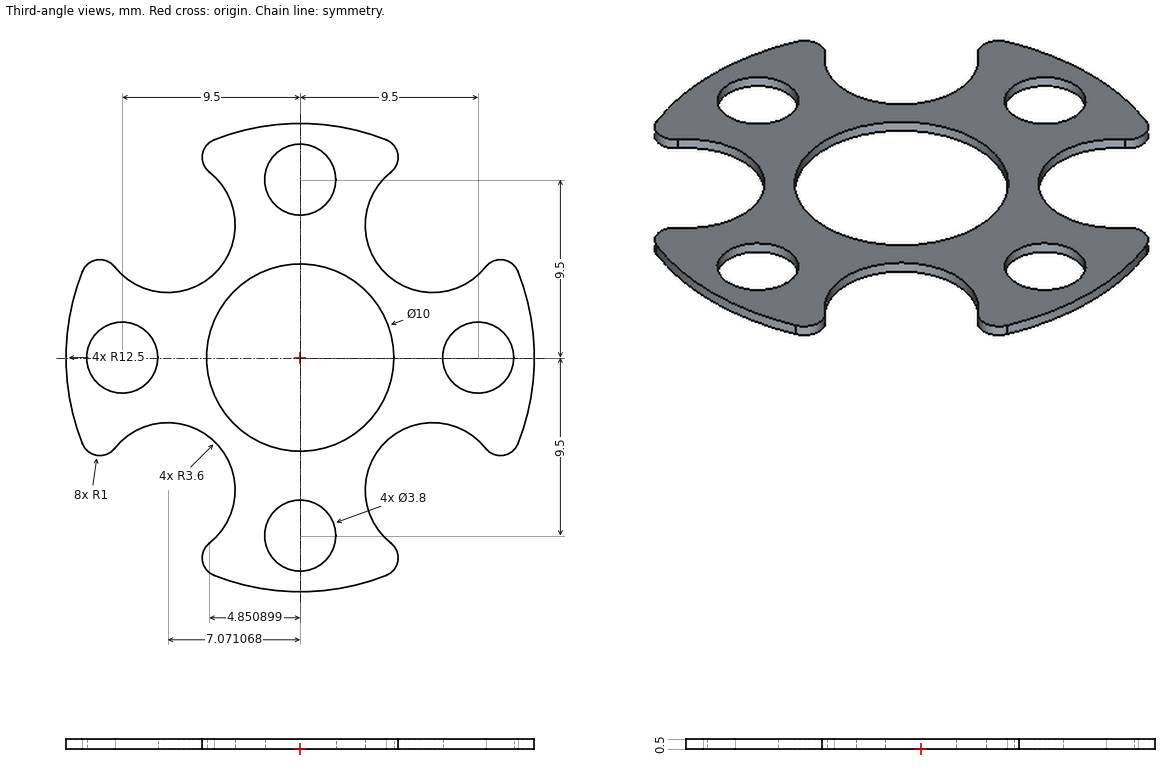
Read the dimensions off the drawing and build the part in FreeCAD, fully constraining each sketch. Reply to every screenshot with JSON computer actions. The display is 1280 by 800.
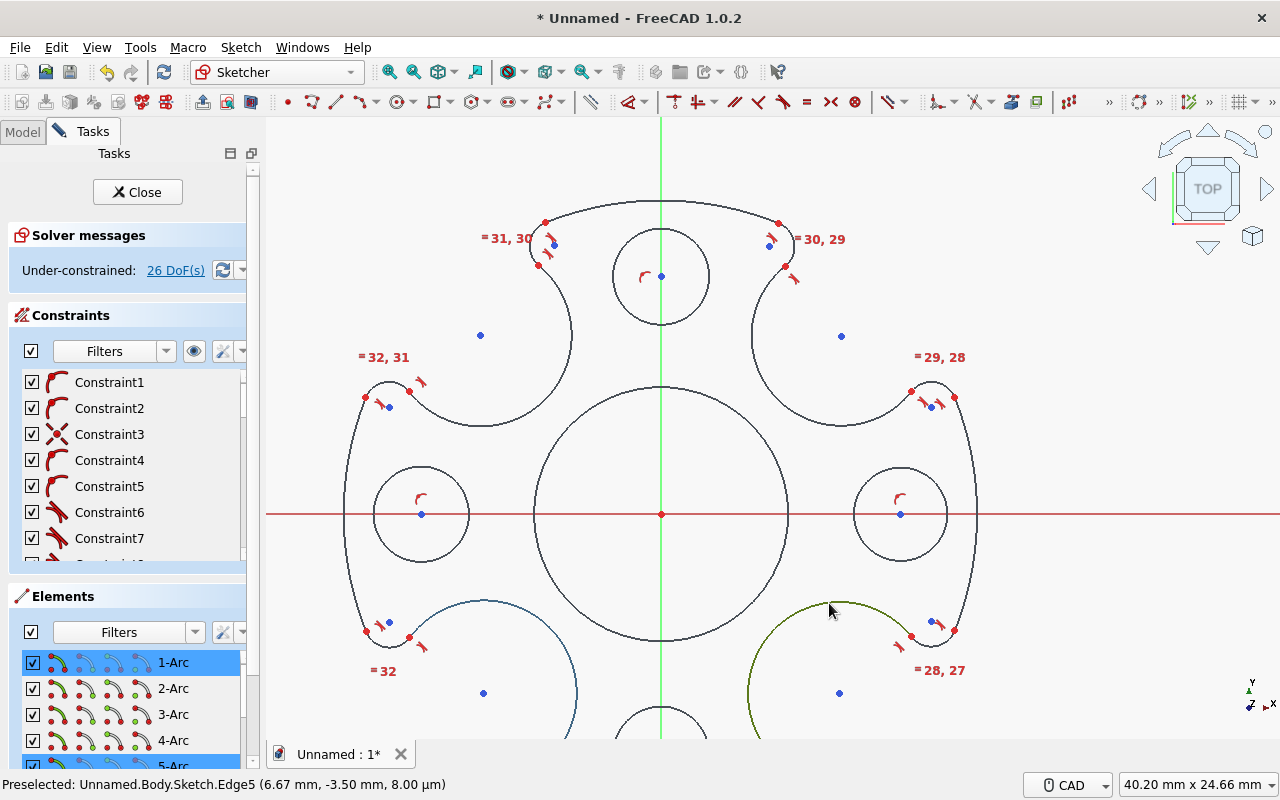
{"action": "left_click", "coordinate": [752, 347]}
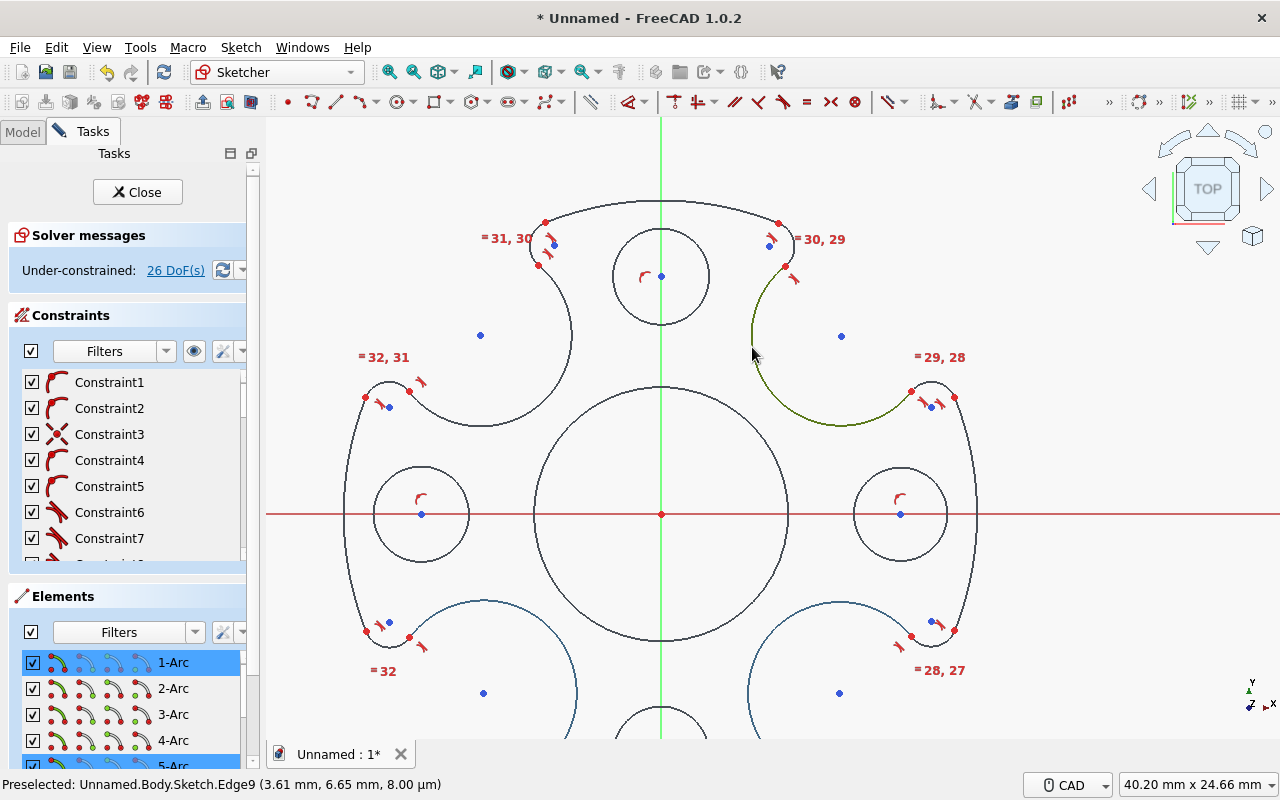
{"action": "left_click", "coordinate": [490, 426]}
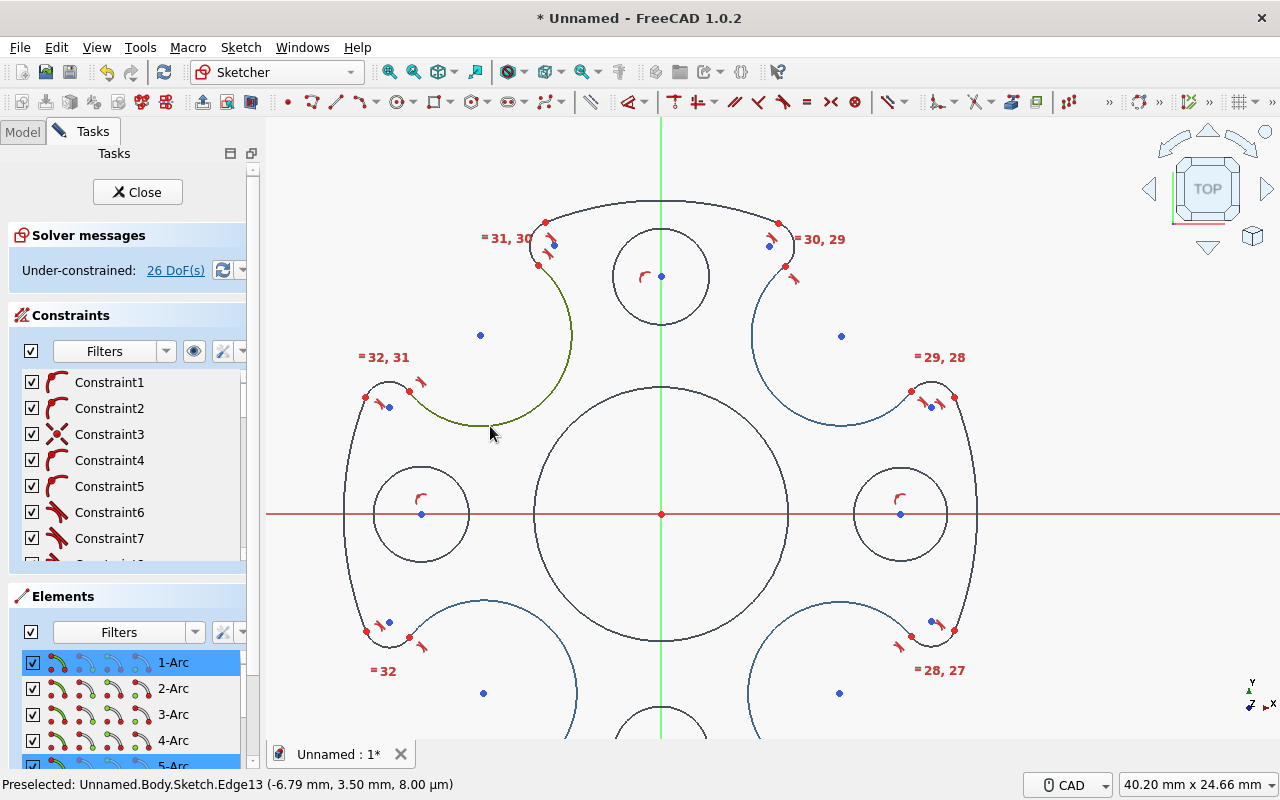
{"action": "key", "text": "e"}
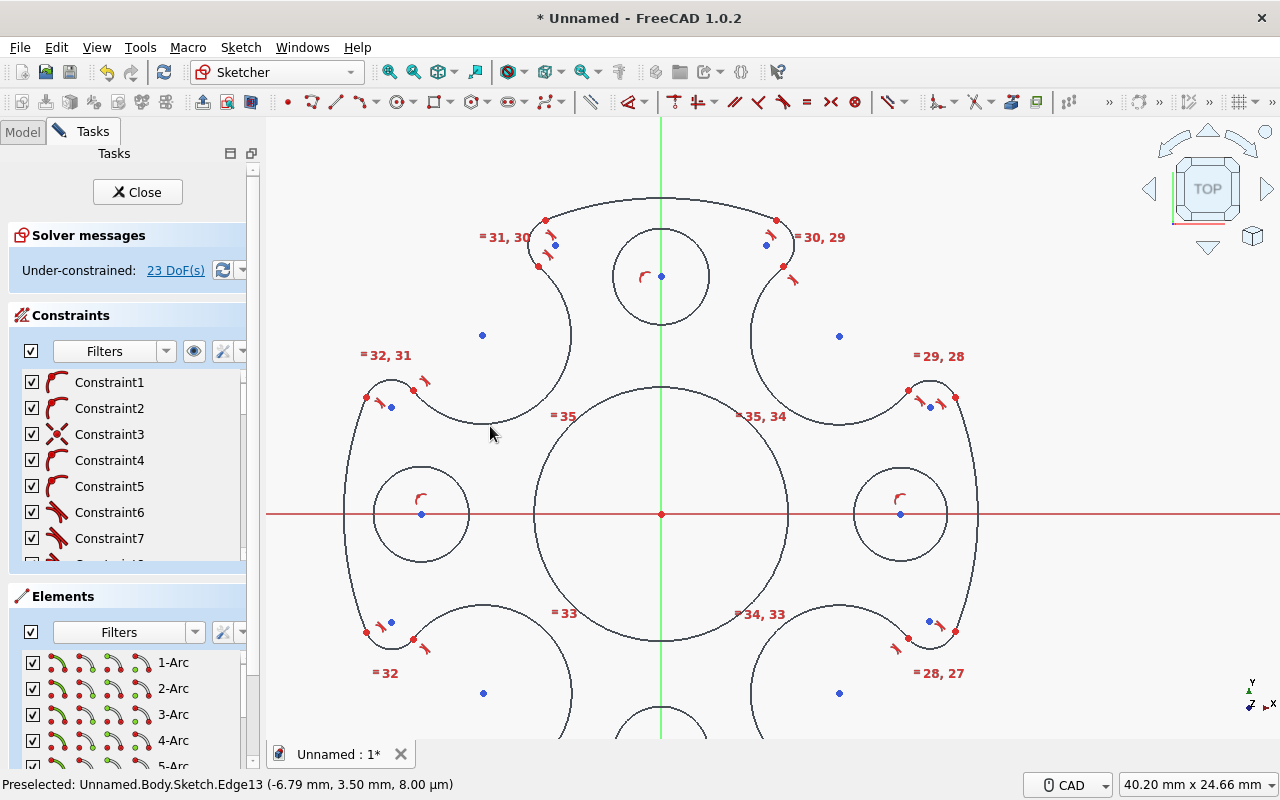
{"action": "scroll", "coordinate": [793, 253], "scroll_direction": "down", "scroll_amount": 2}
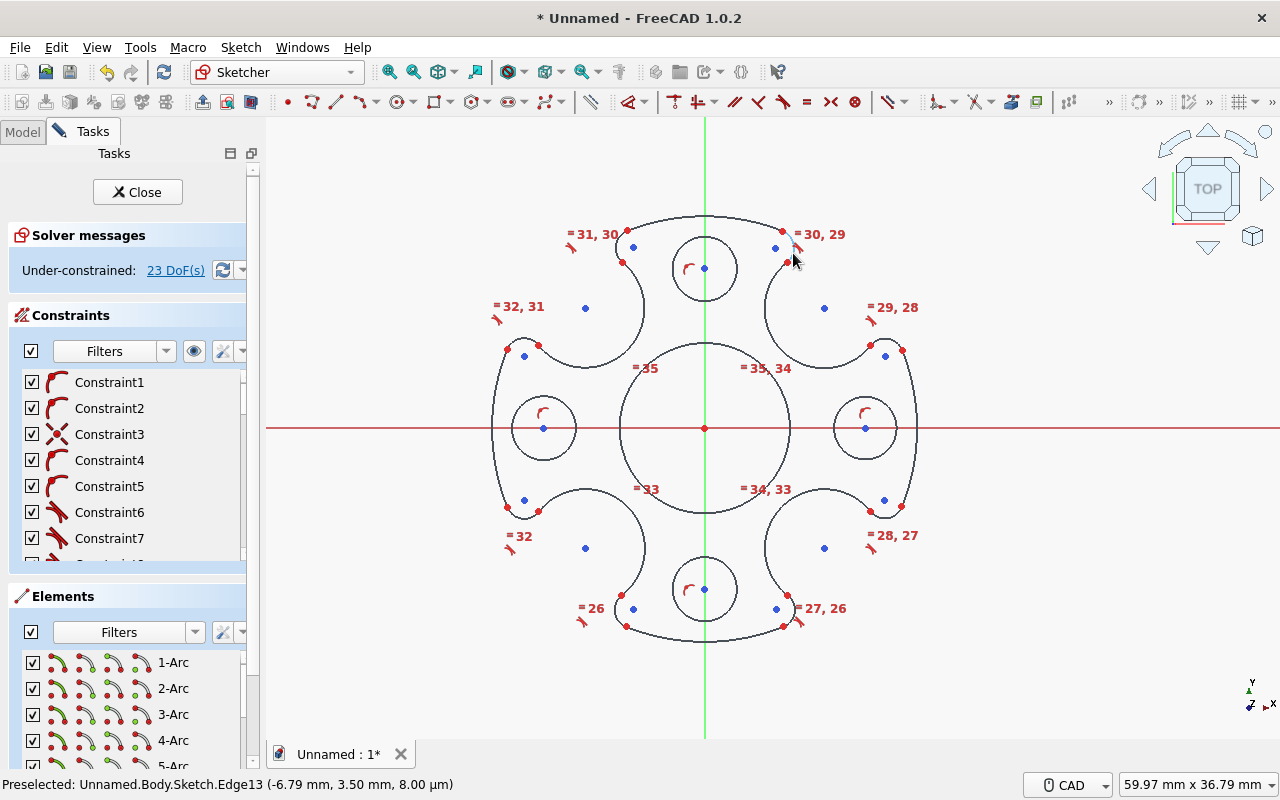
{"action": "left_click", "coordinate": [673, 639]}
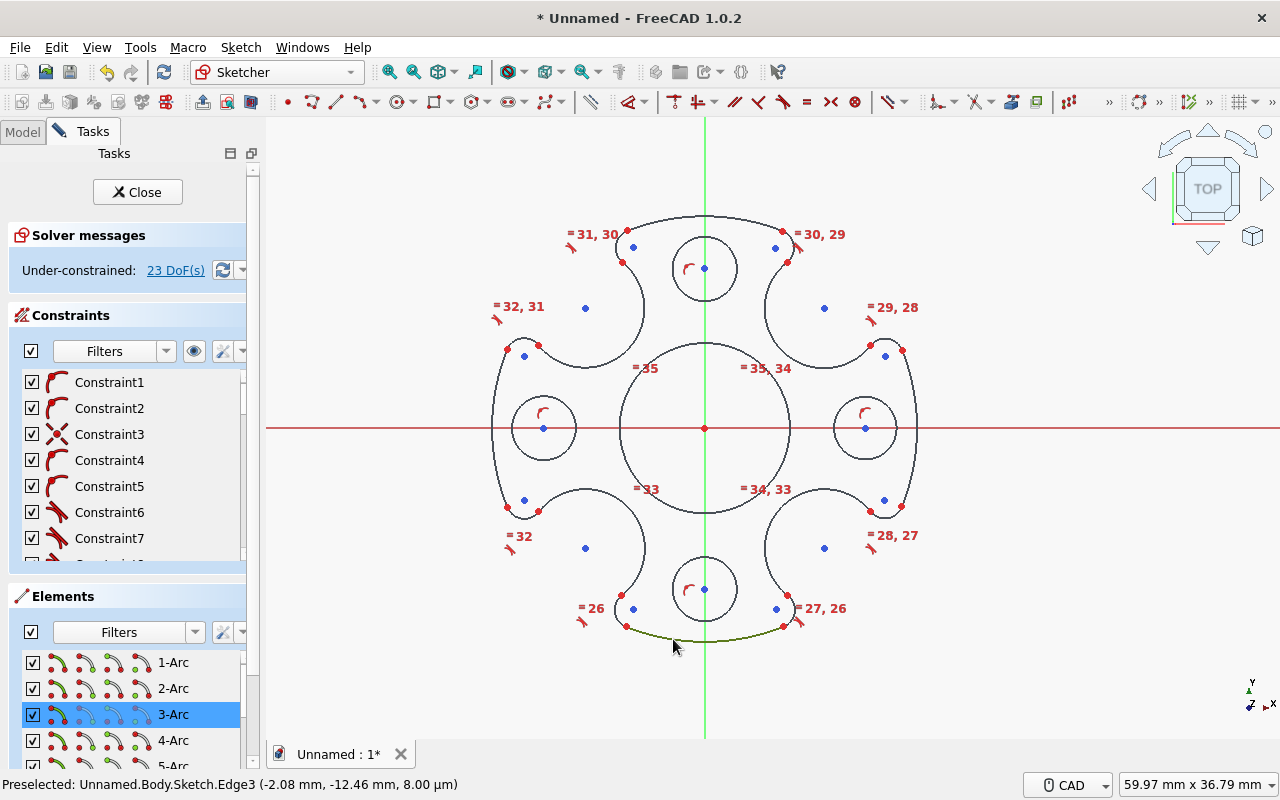
{"action": "left_click", "coordinate": [915, 460]}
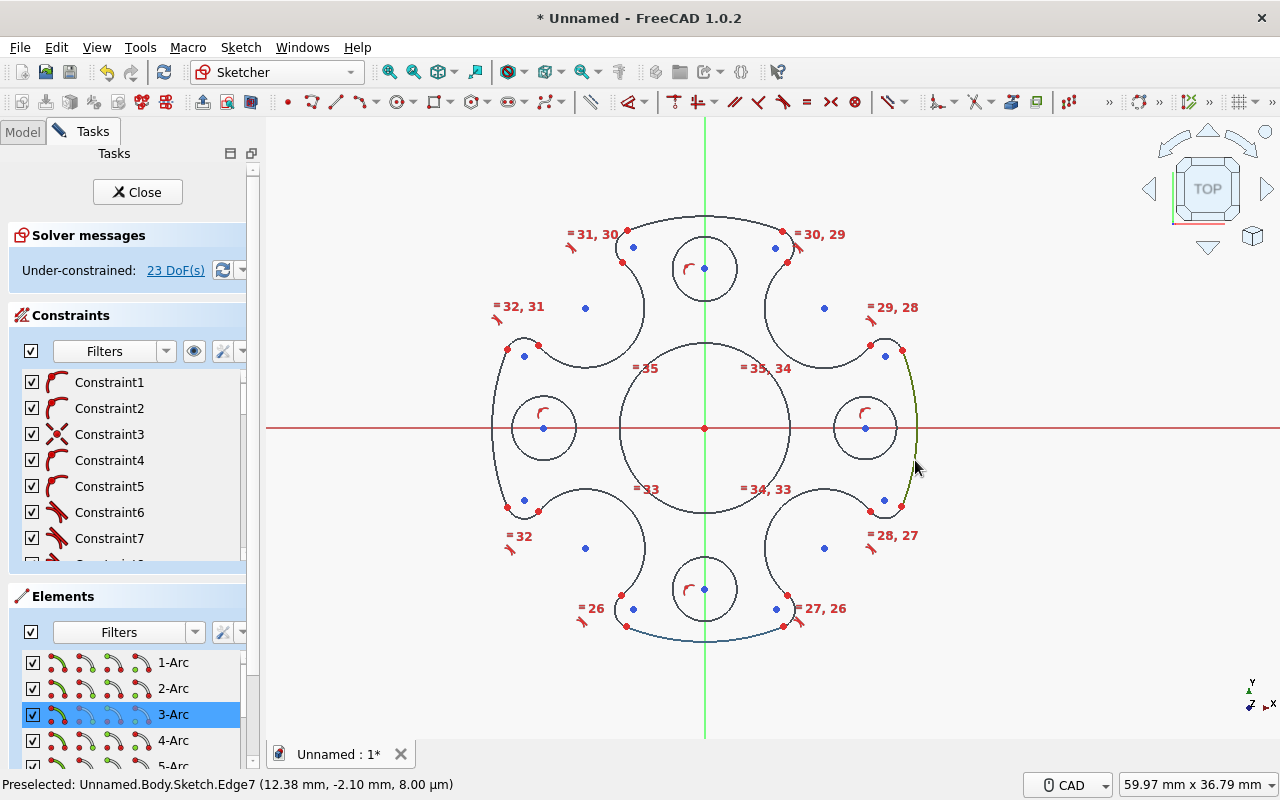
{"action": "left_click", "coordinate": [736, 219]}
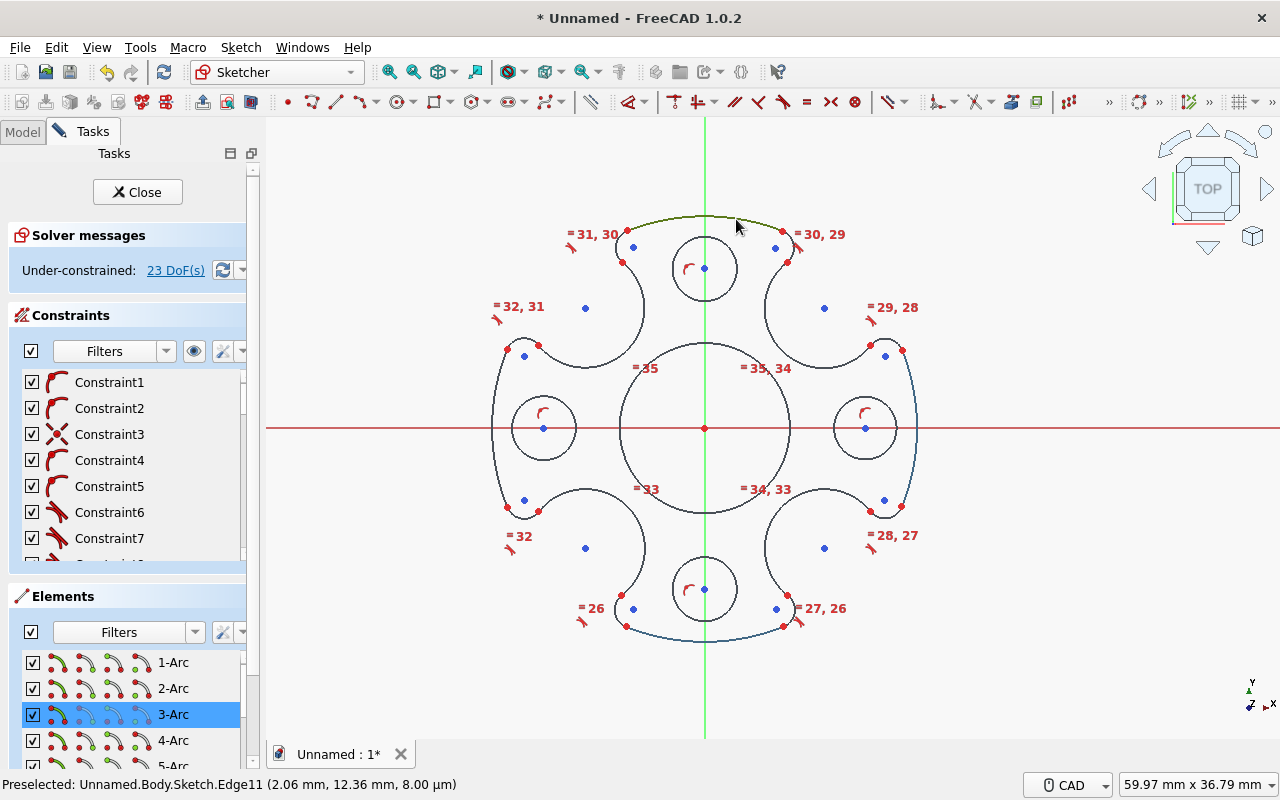
{"action": "left_click", "coordinate": [495, 396]}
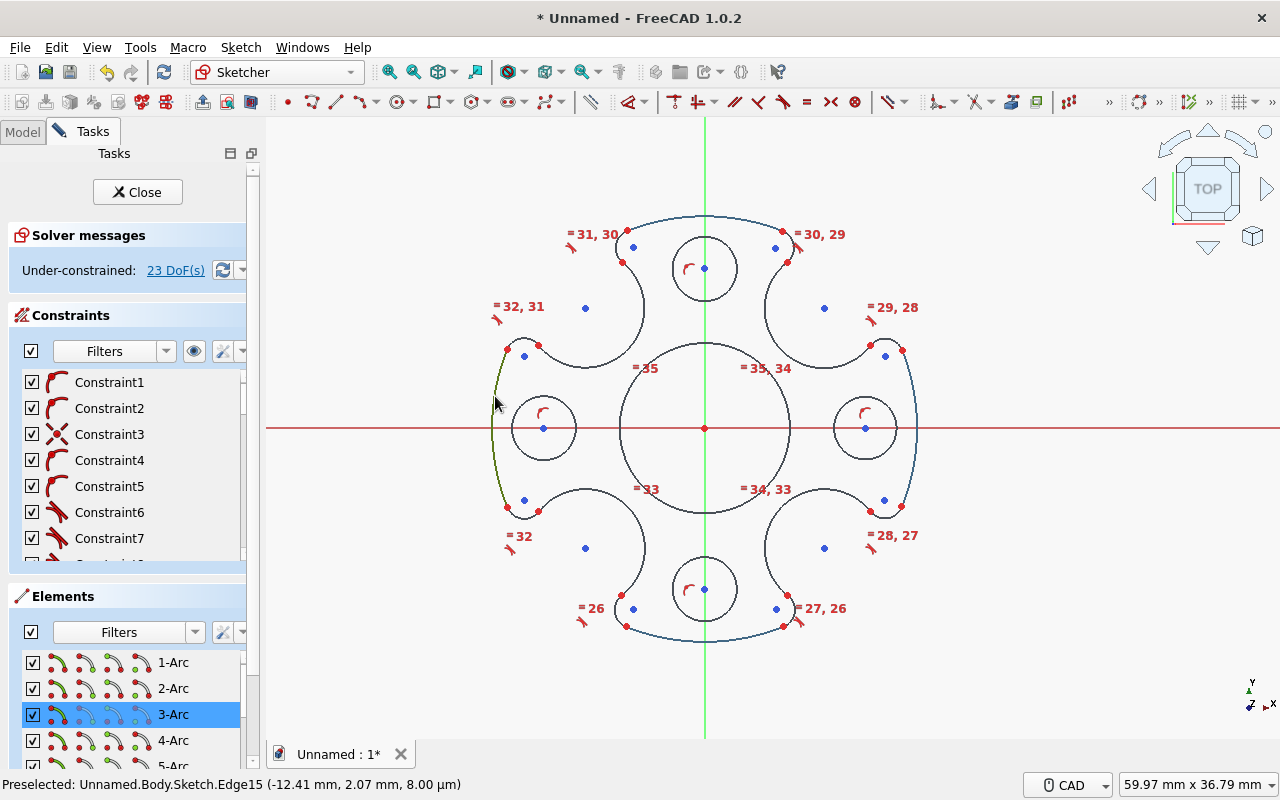
{"action": "left_click", "coordinate": [808, 102]}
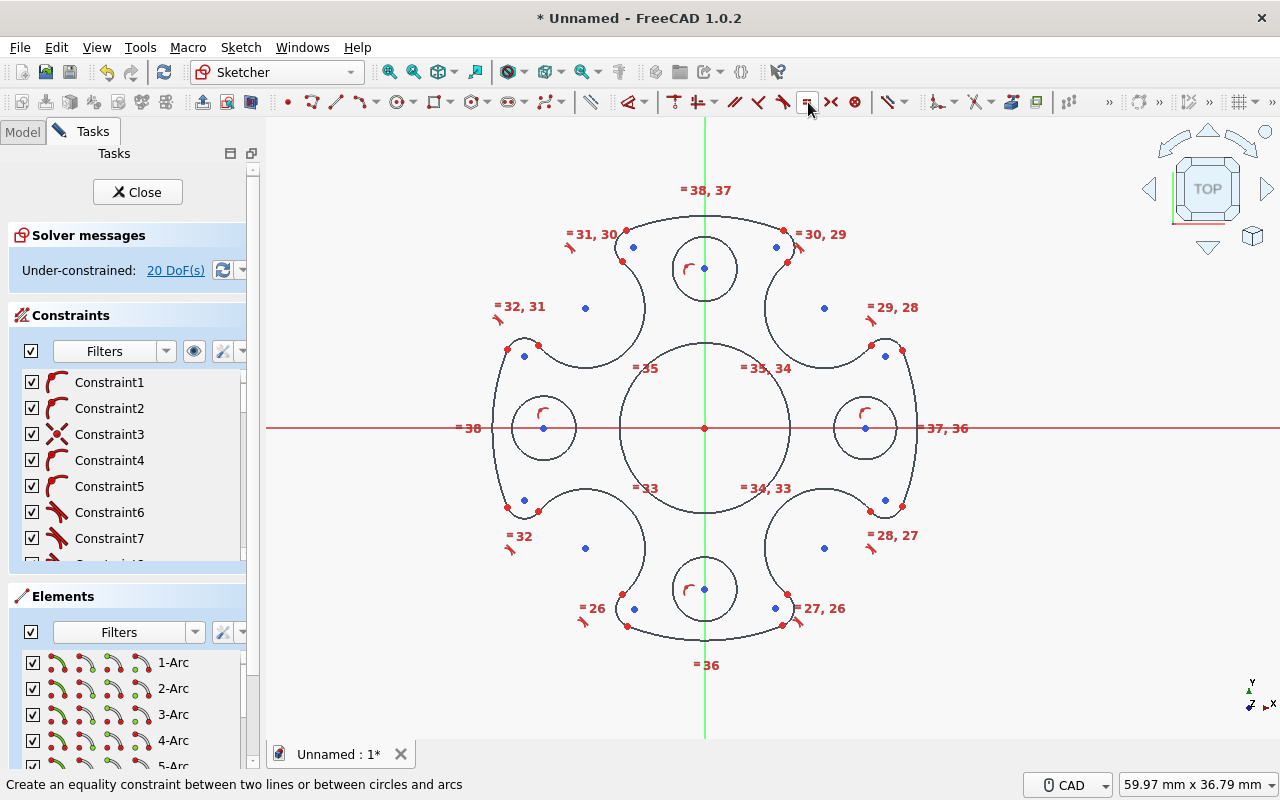
{"action": "left_click", "coordinate": [727, 566]}